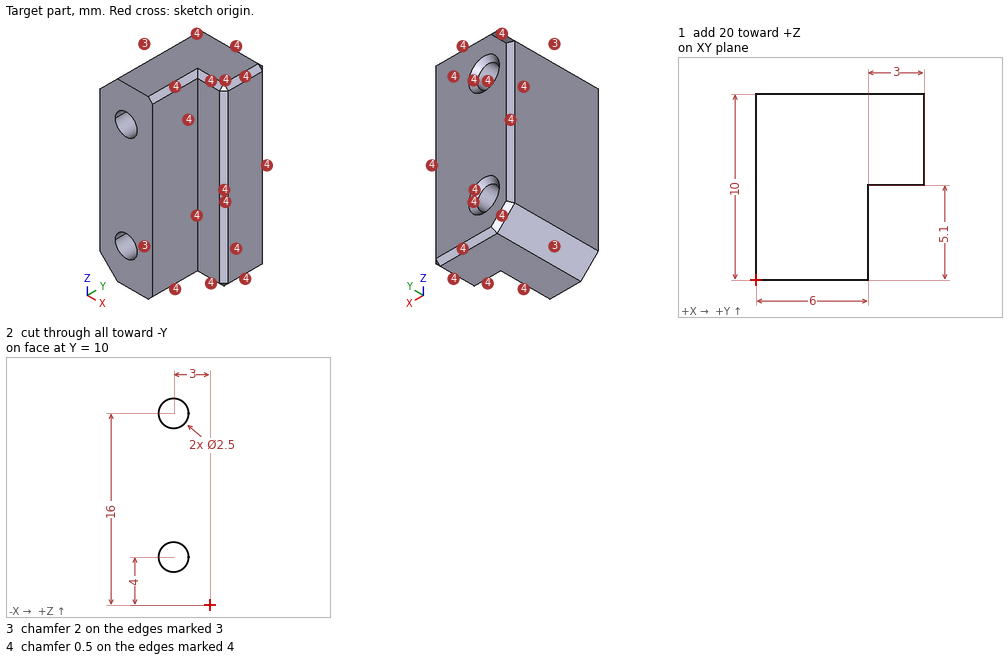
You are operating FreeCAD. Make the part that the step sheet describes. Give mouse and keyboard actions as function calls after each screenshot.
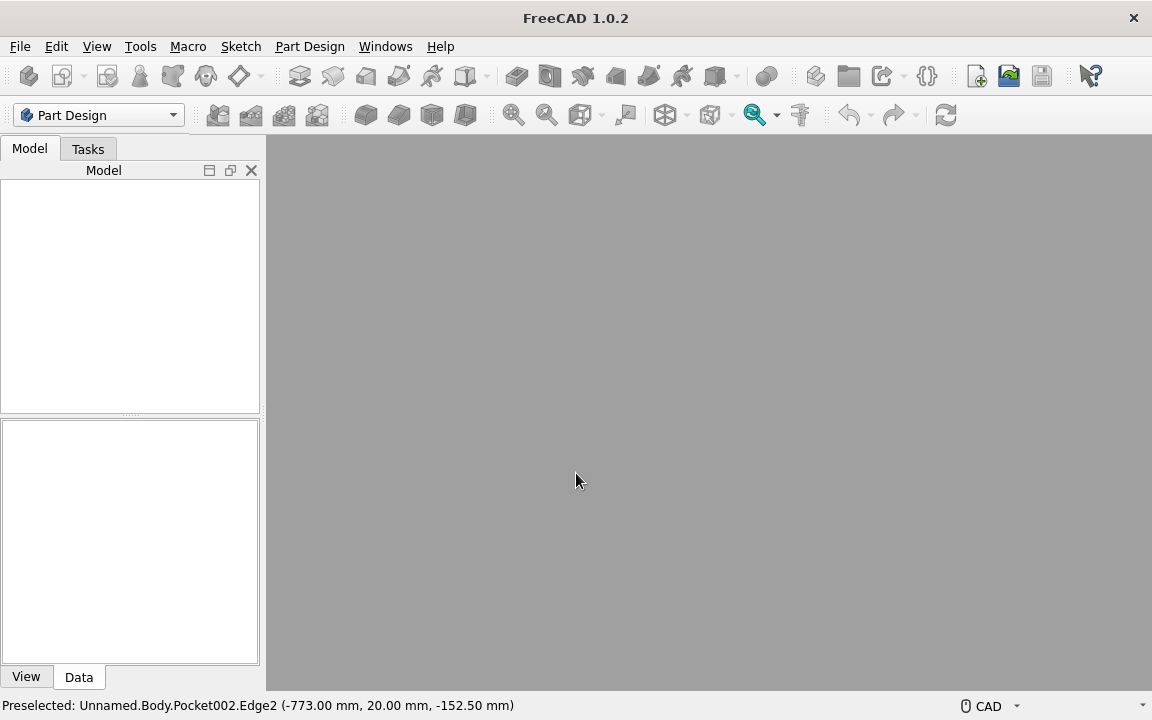
click(976, 76)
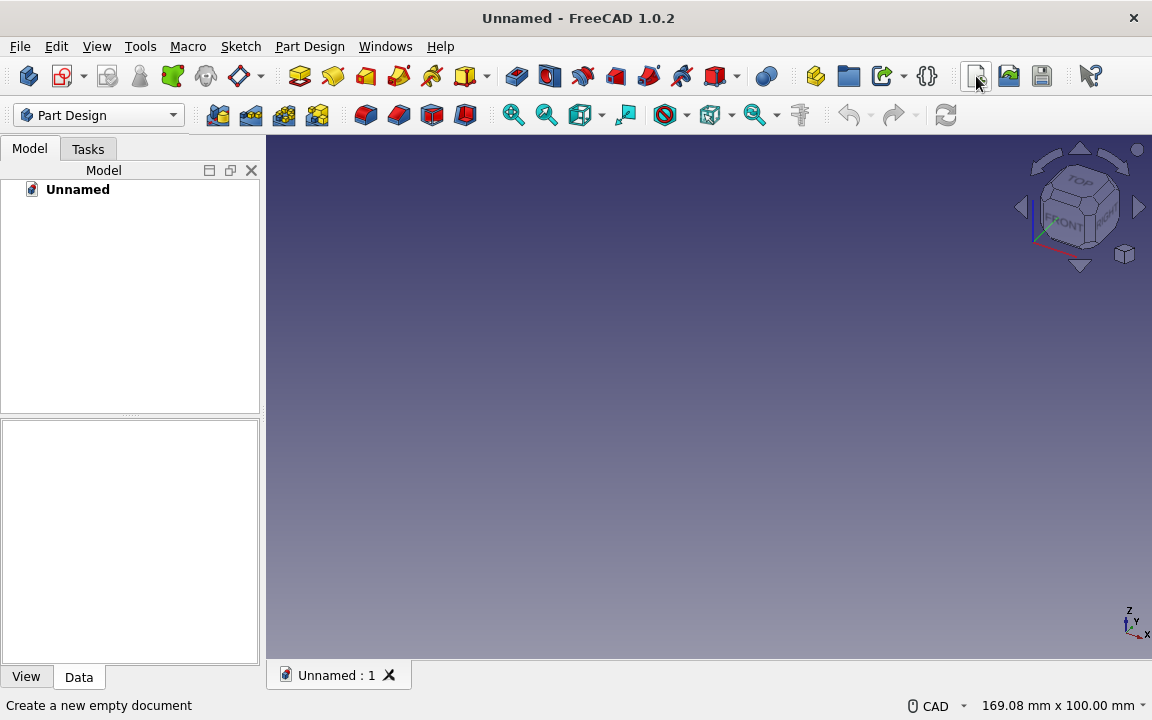
click(62, 76)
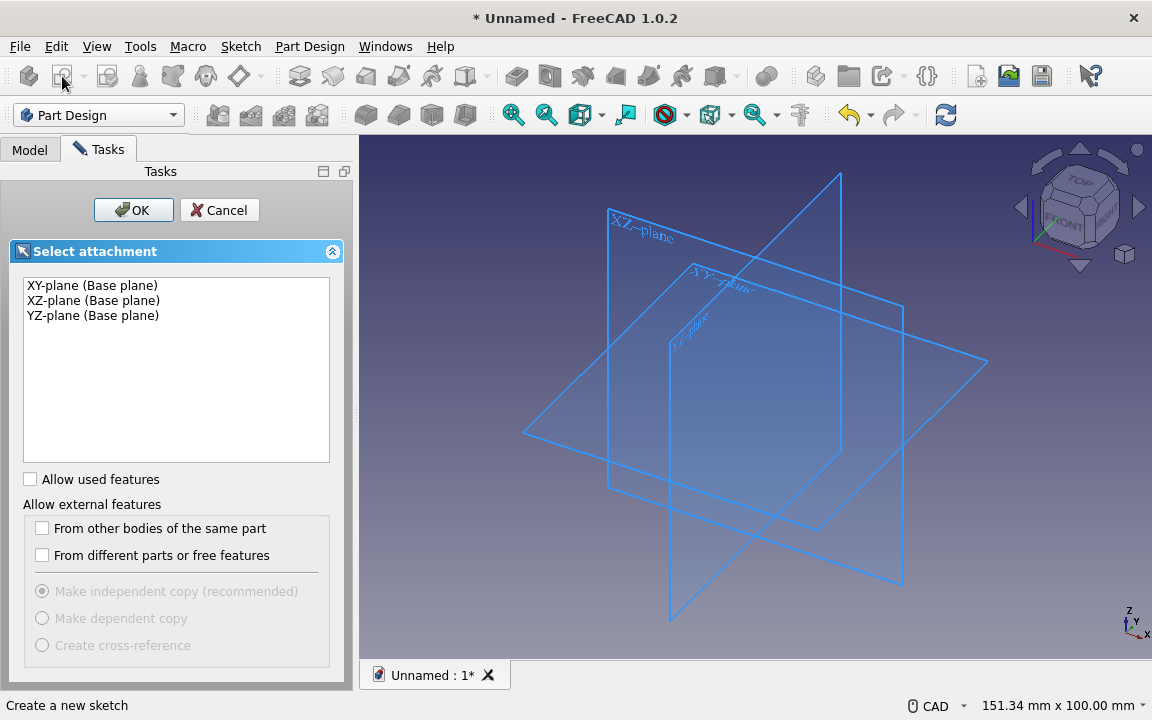
click(84, 286)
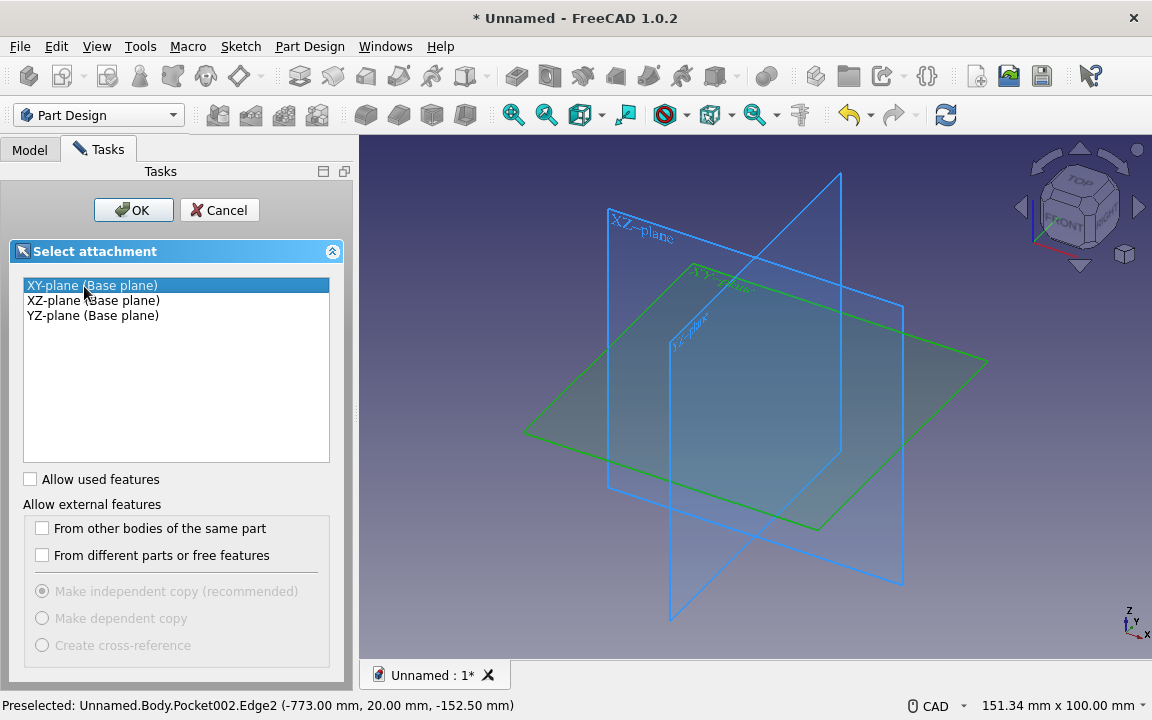
click(134, 210)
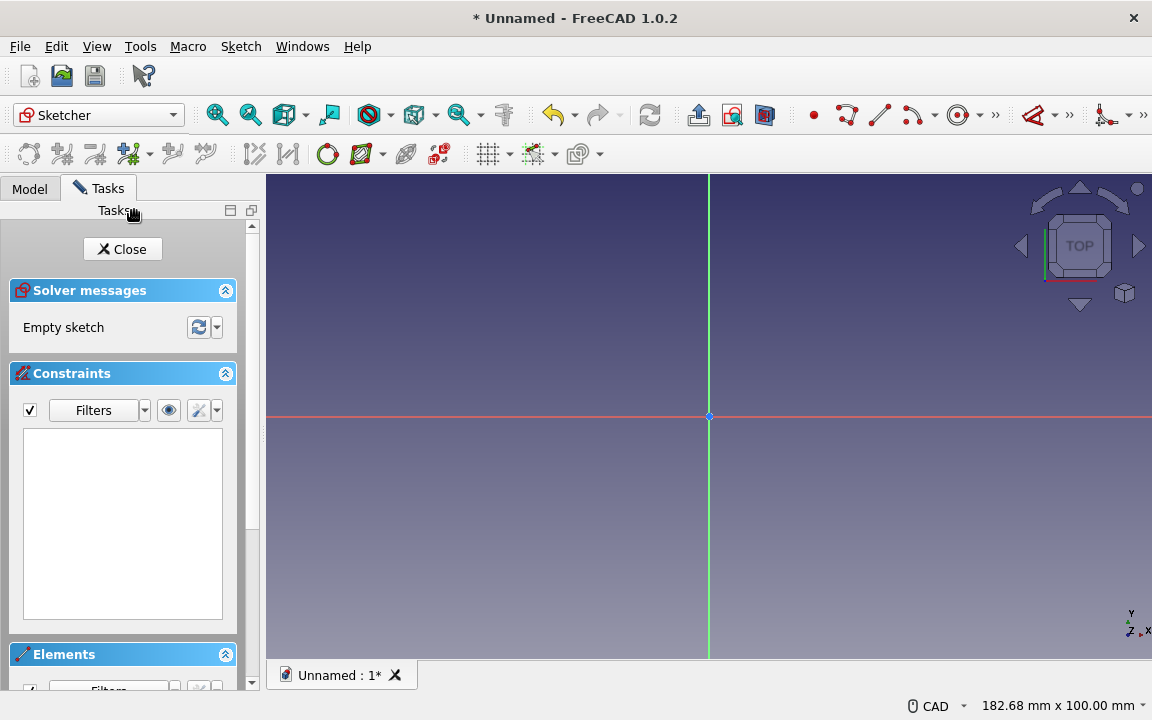
scroll(749, 387, up, 9)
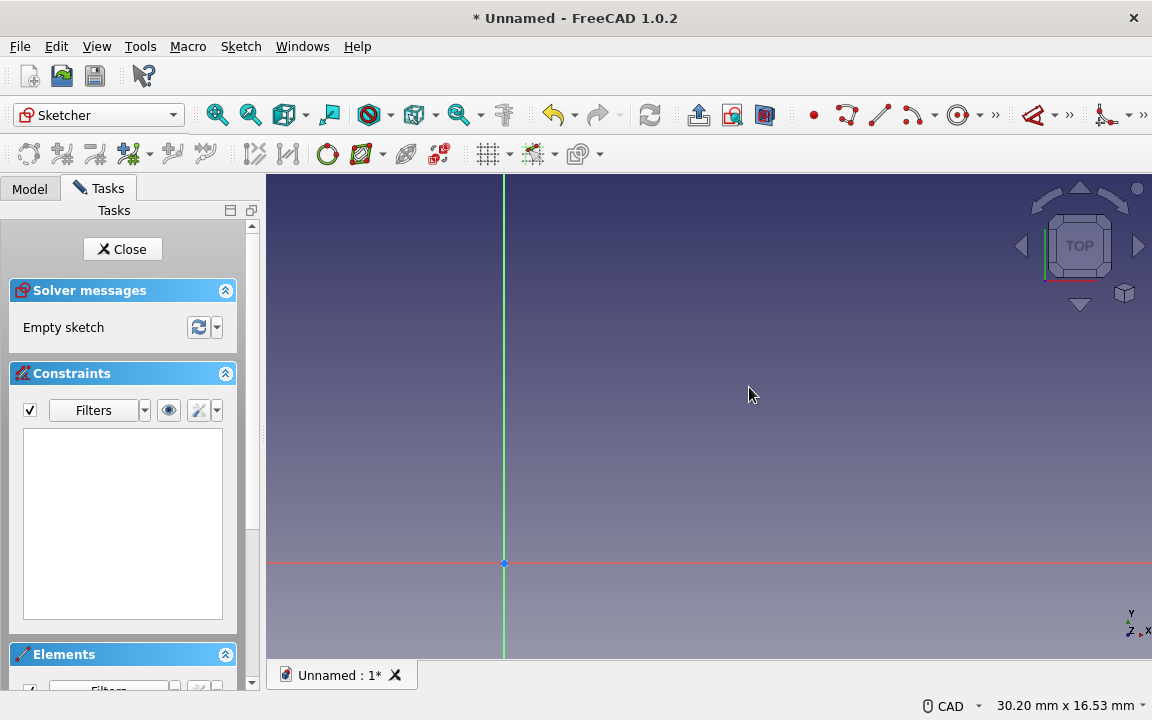
click(847, 116)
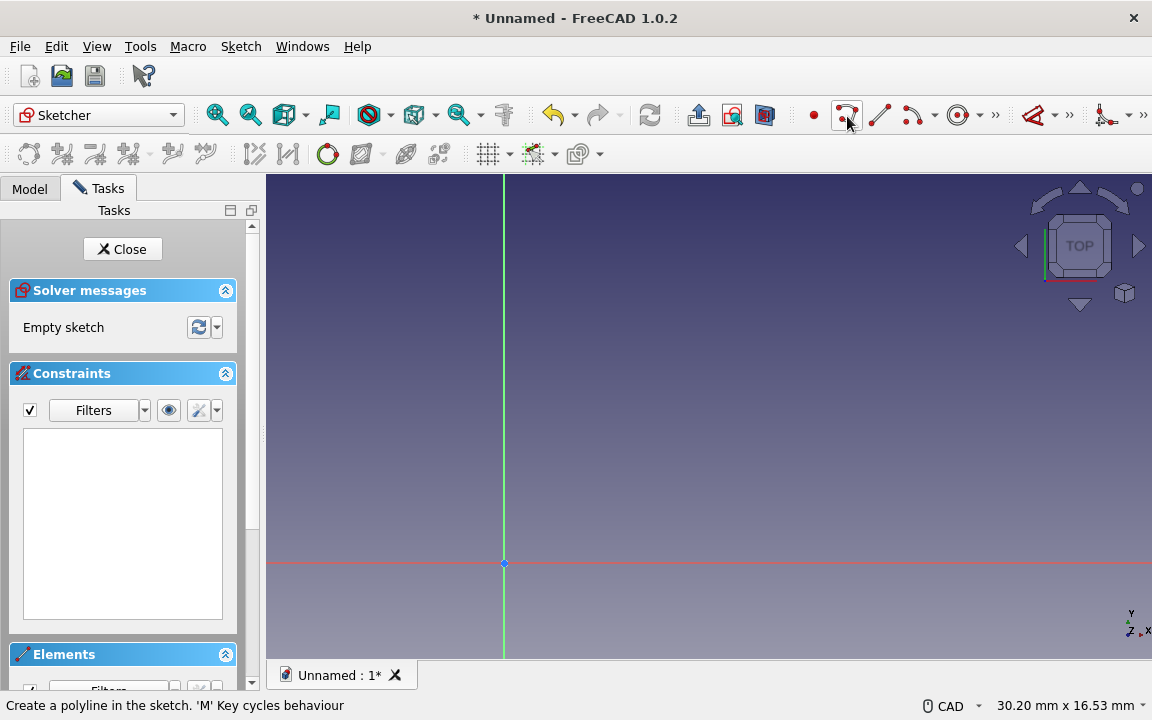
click(504, 563)
click(680, 554)
click(680, 414)
click(768, 414)
click(768, 270)
click(513, 270)
click(504, 563)
key(Escape)
key(Escape)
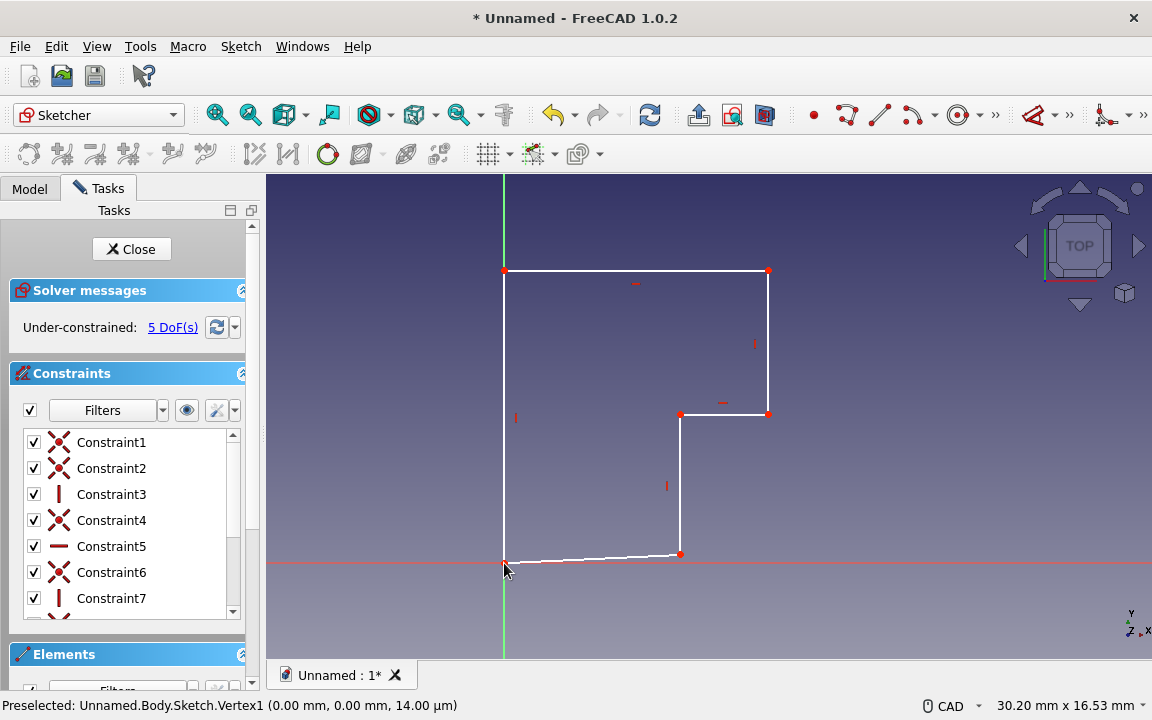
click(557, 561)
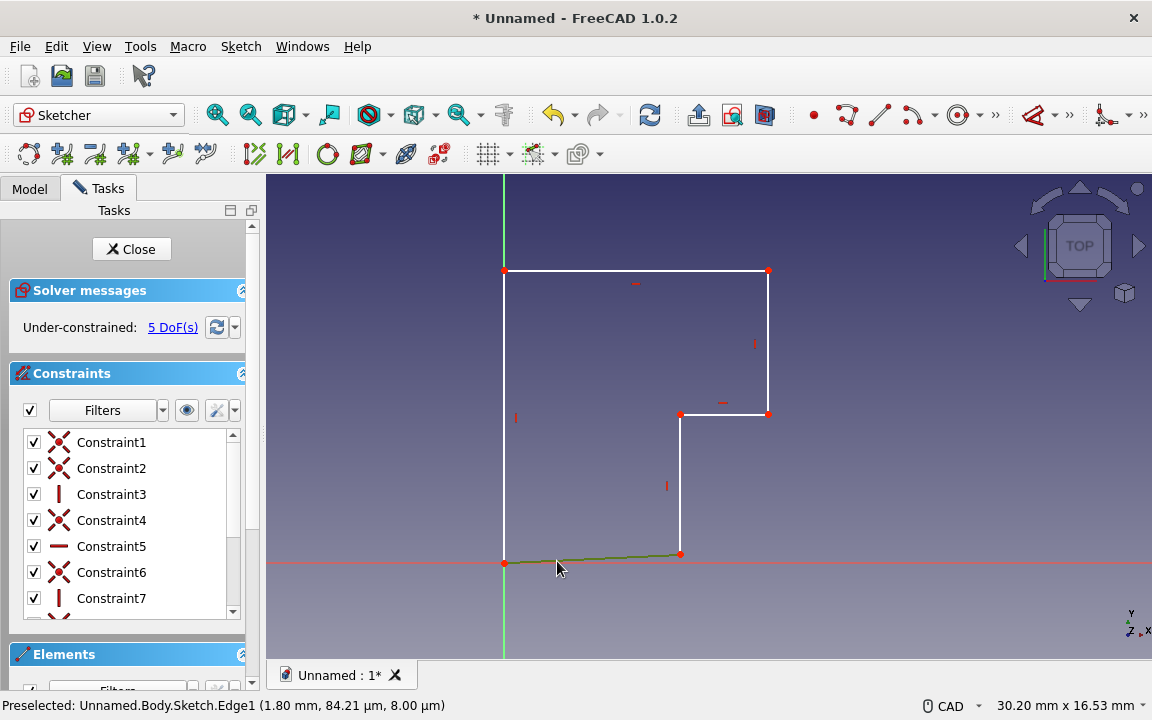
key(h)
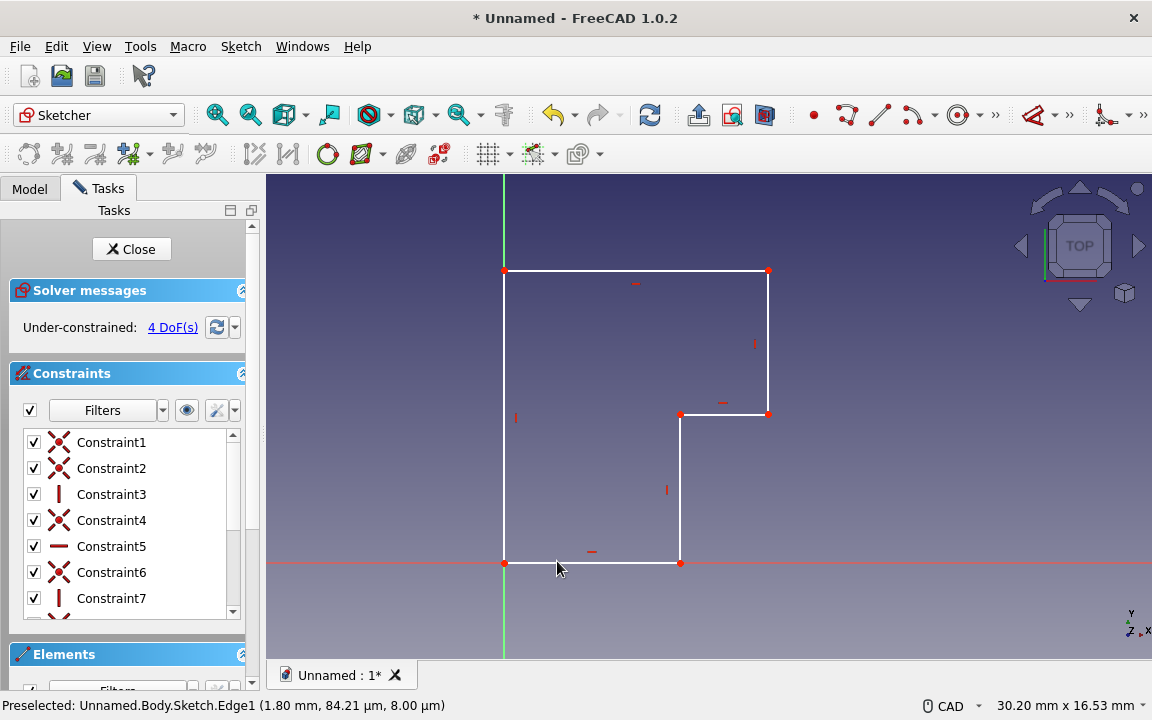
click(1032, 116)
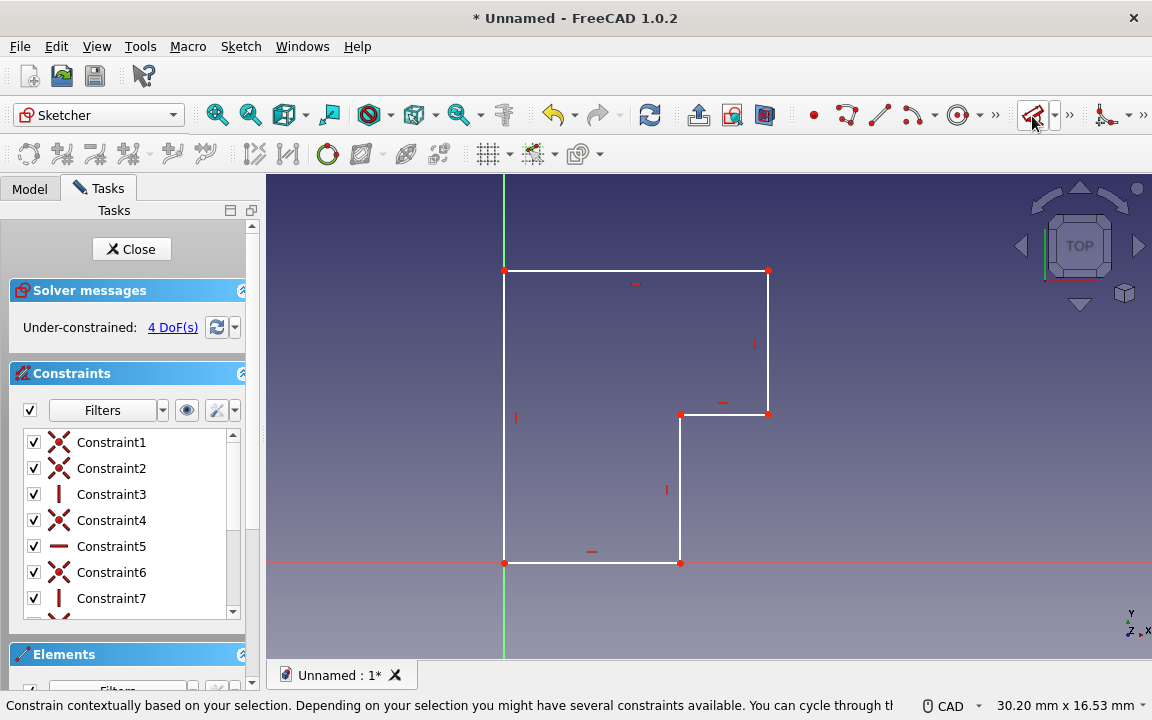
click(557, 563)
click(592, 597)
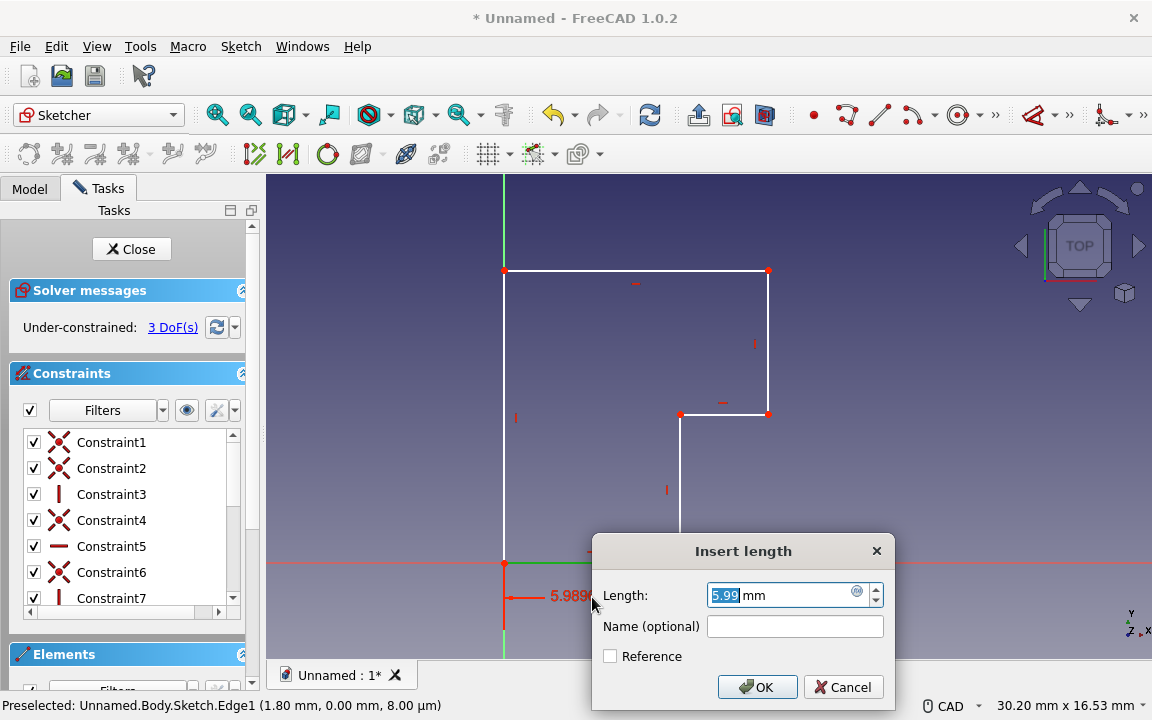
text(6)
key(Return)